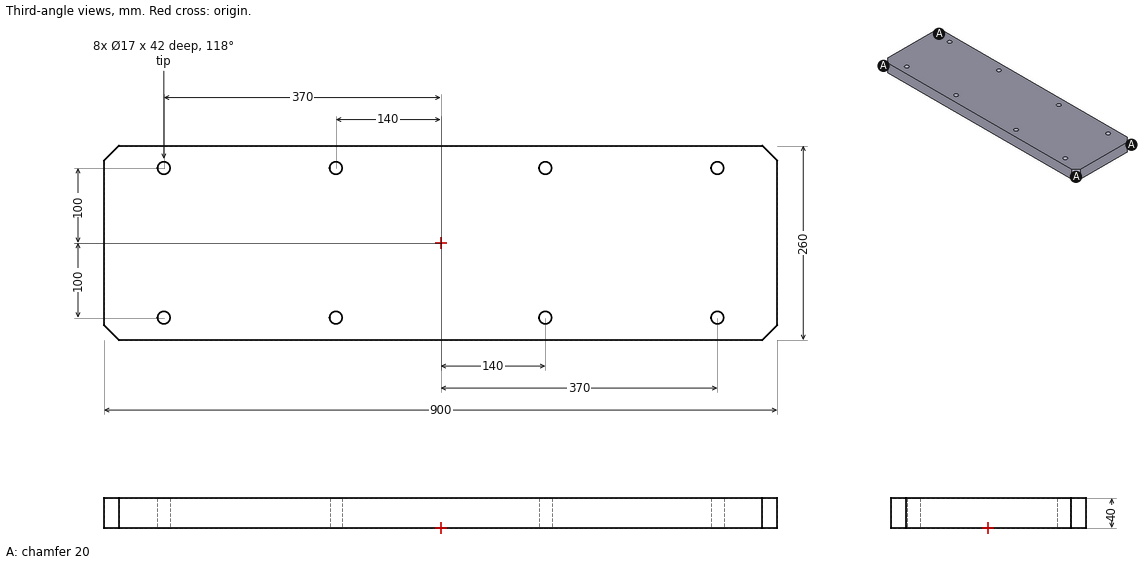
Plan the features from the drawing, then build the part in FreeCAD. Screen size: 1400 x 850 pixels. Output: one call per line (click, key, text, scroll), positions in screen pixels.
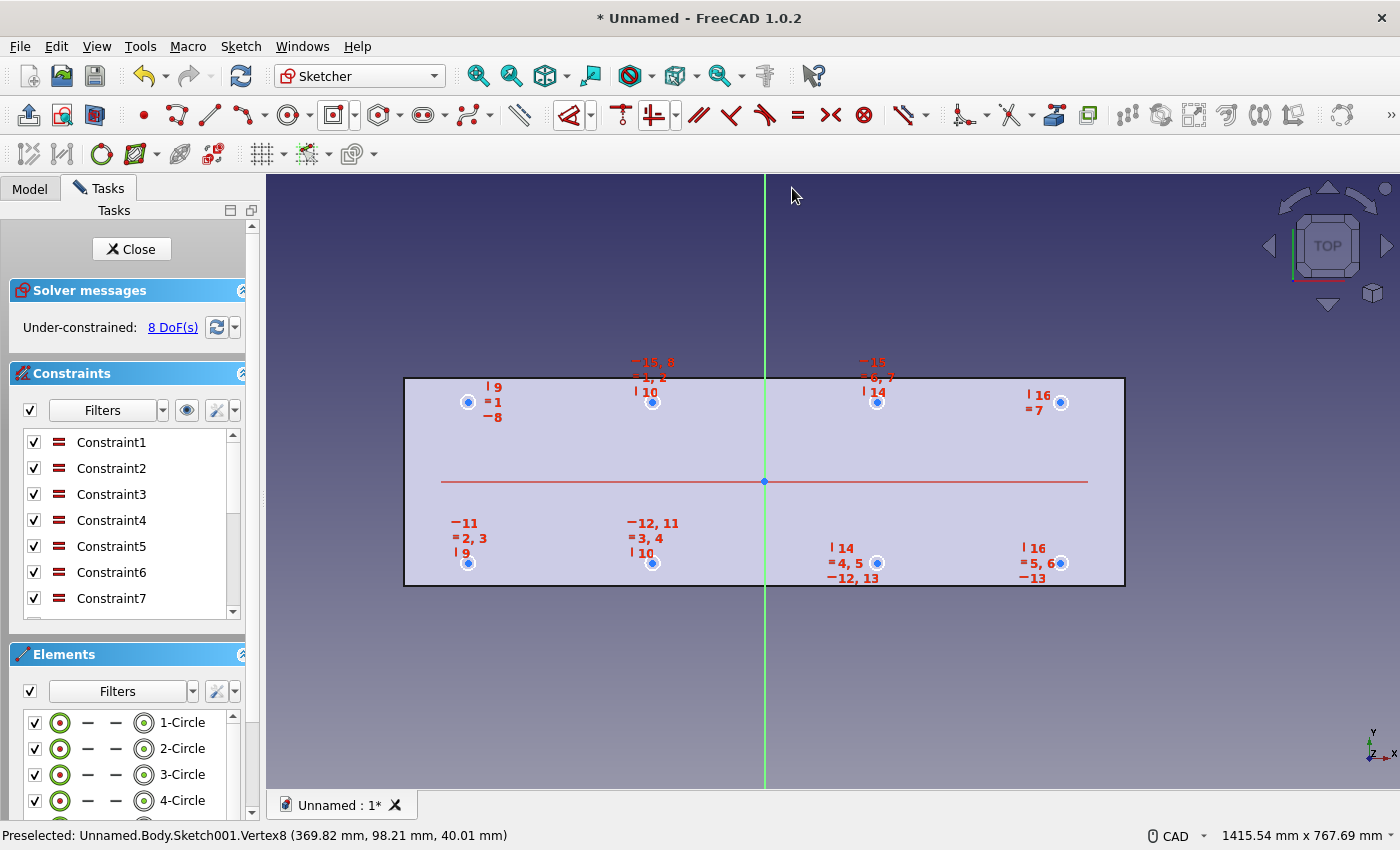
click(877, 402)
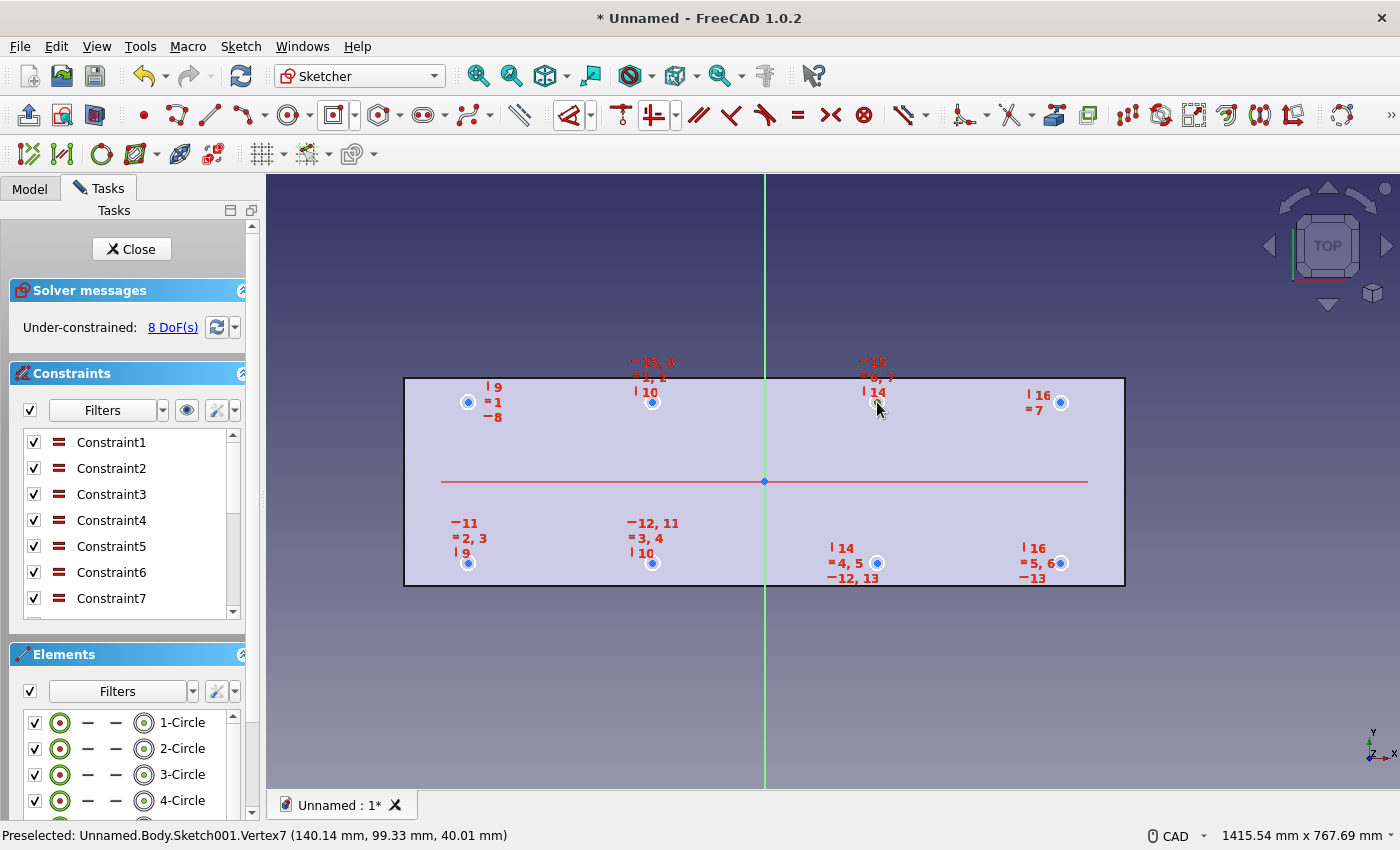
click(1061, 403)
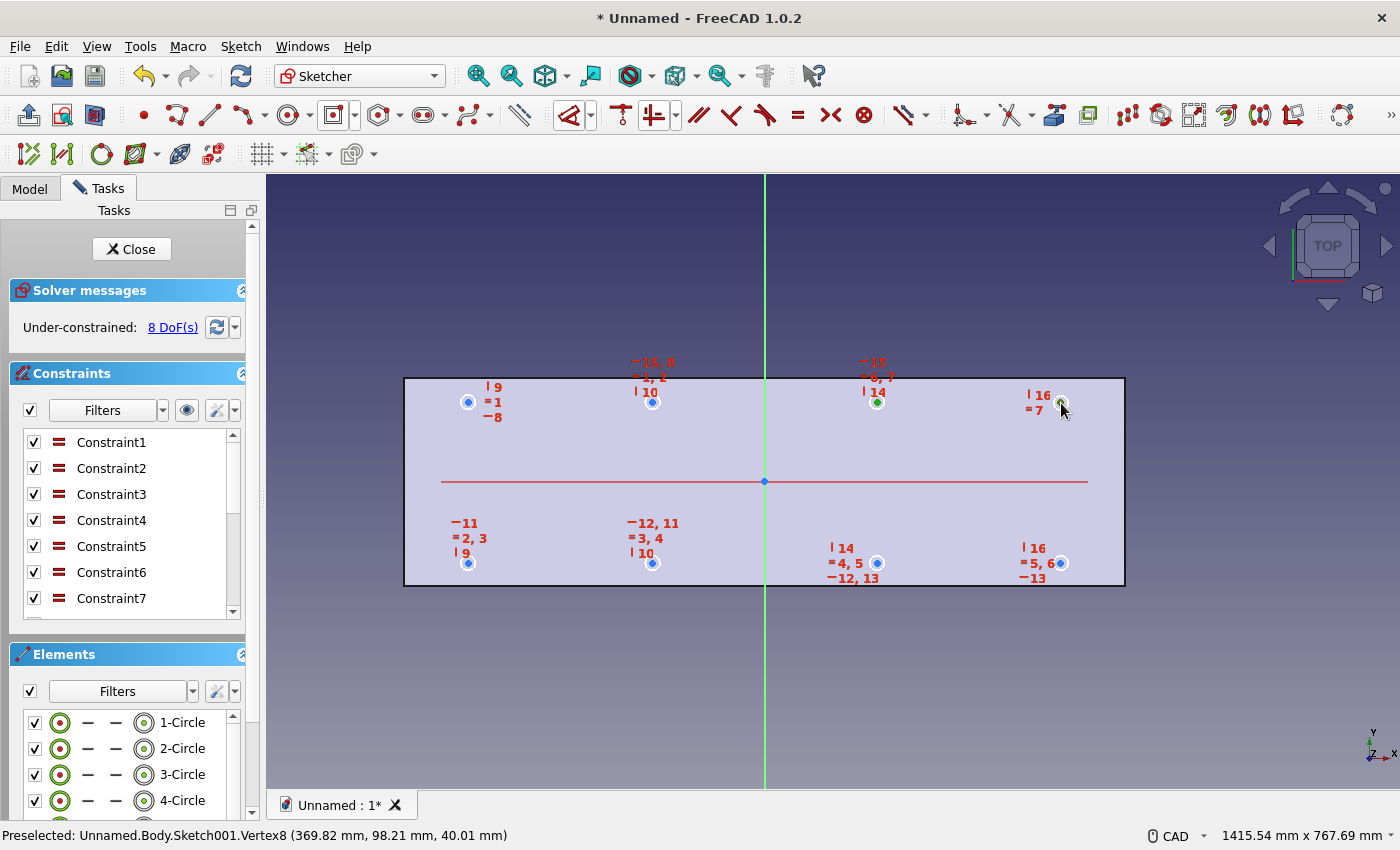
key(h)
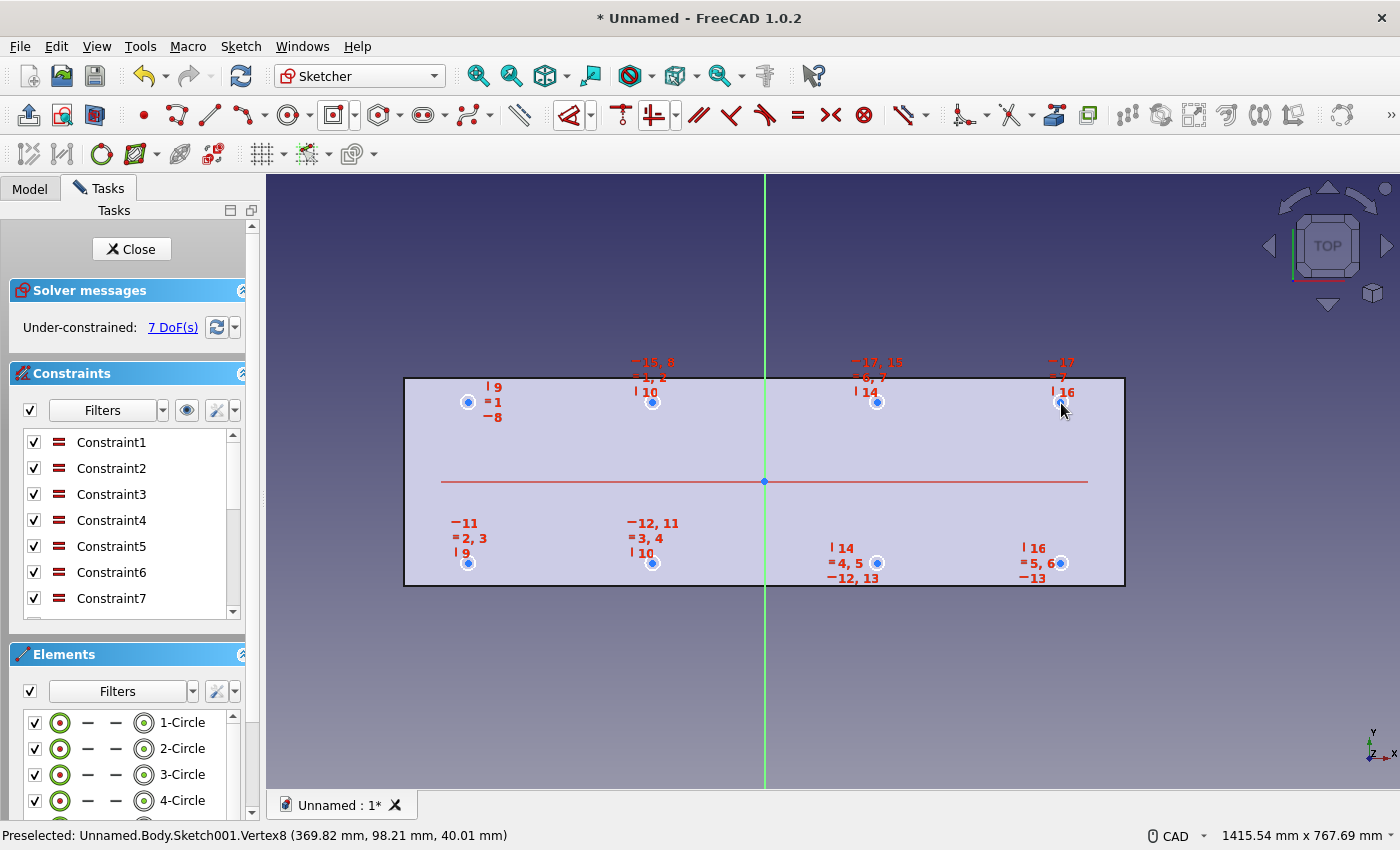
scroll(468, 395, up, 6)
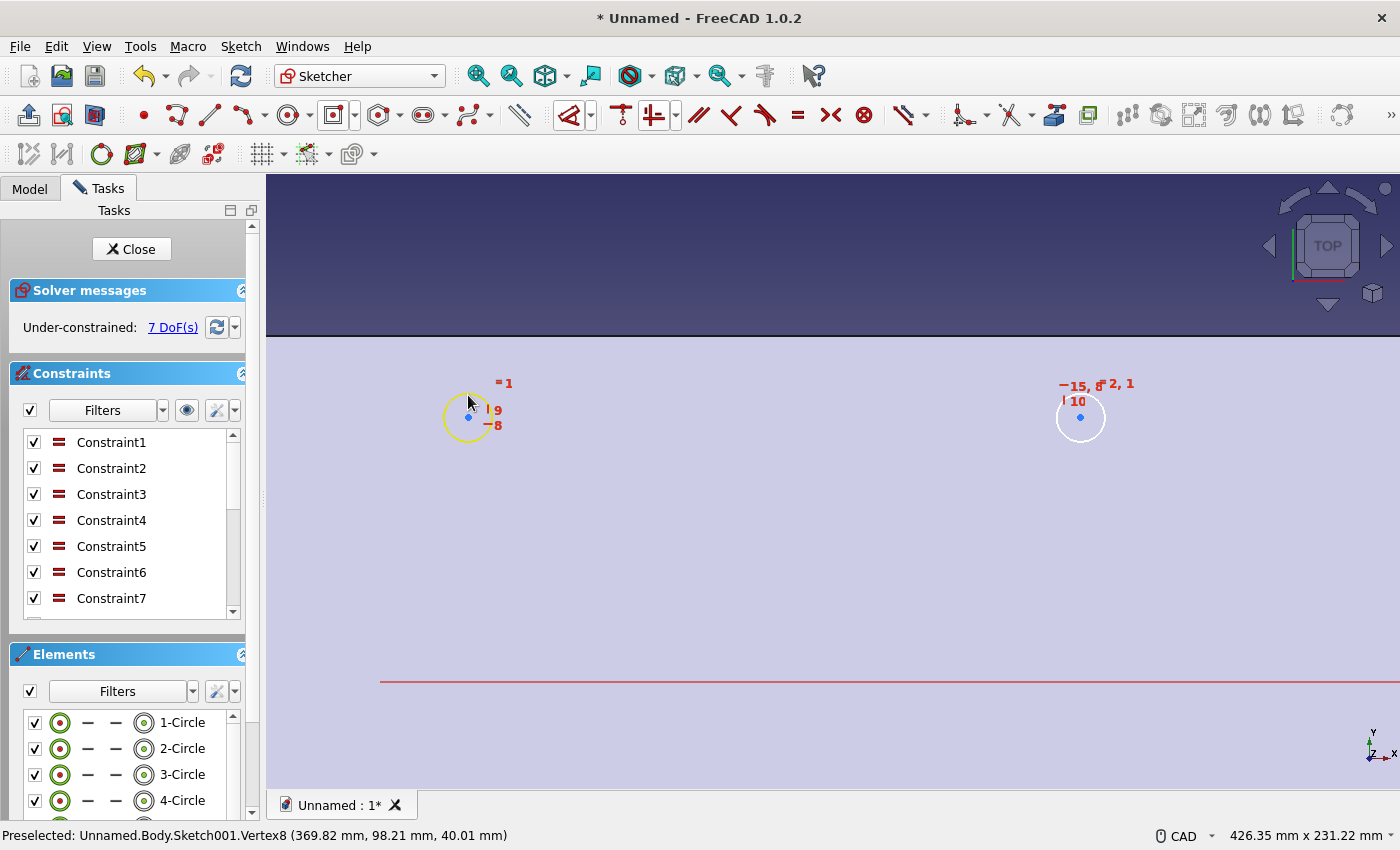
click(469, 394)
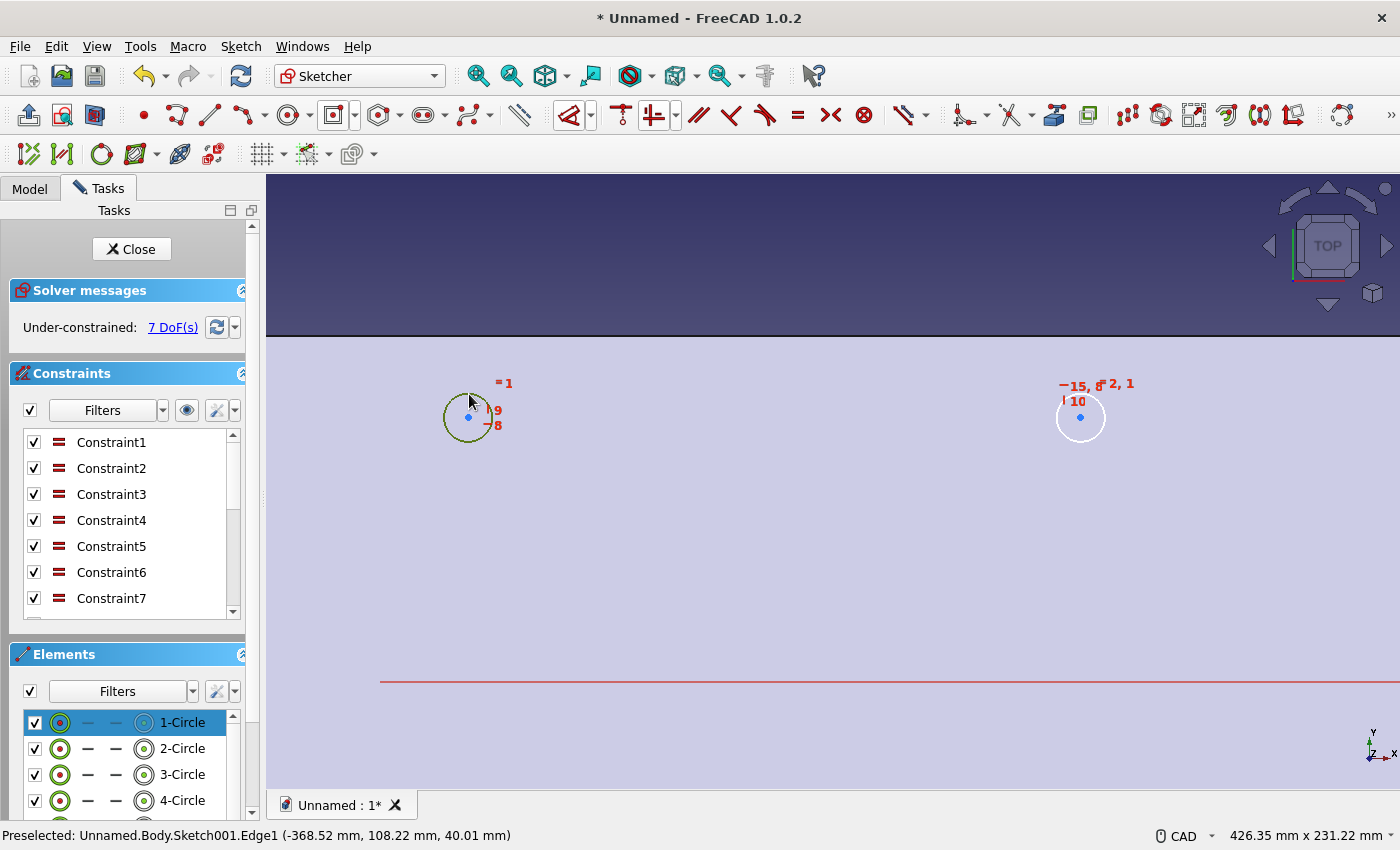
click(590, 116)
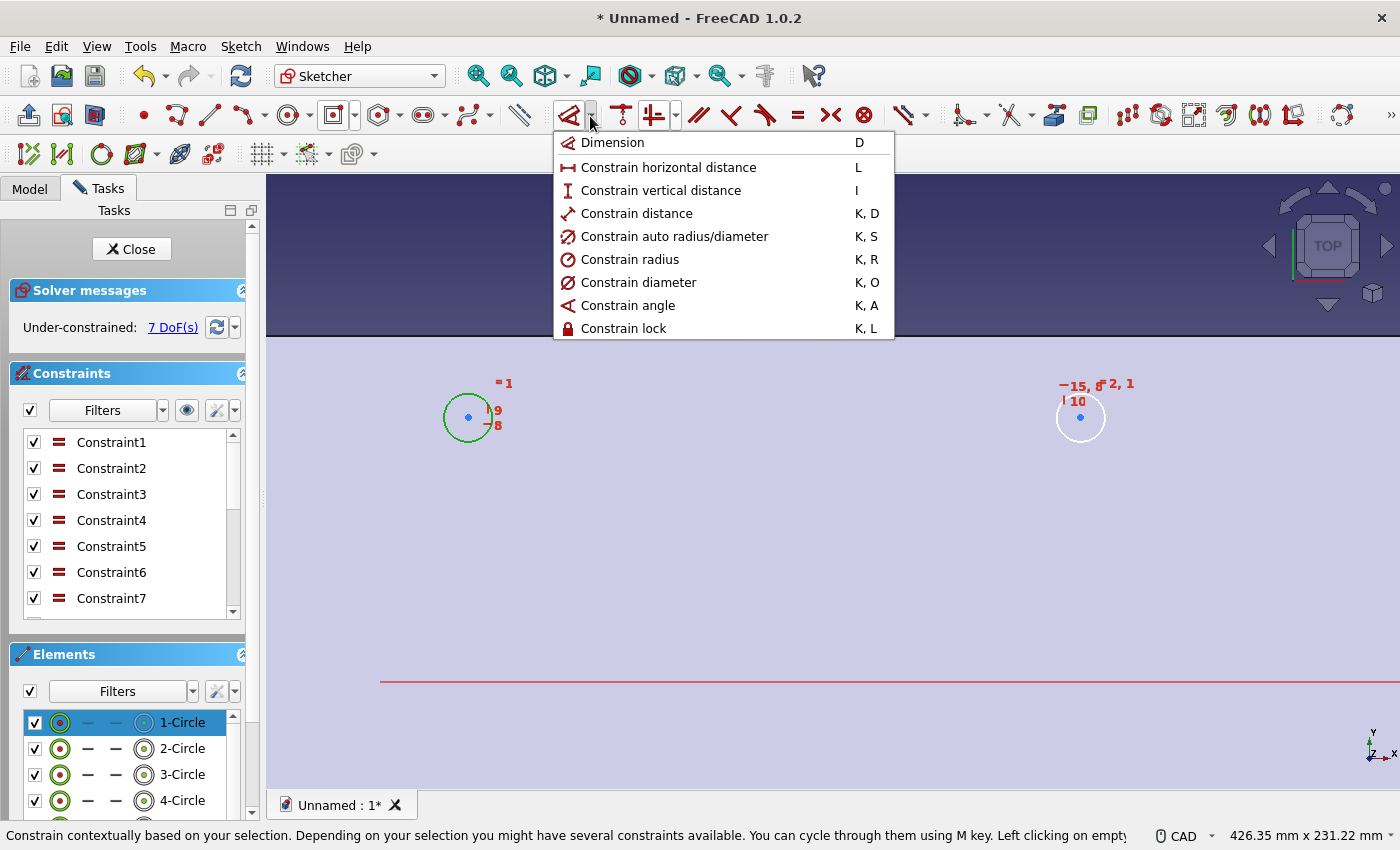
click(724, 282)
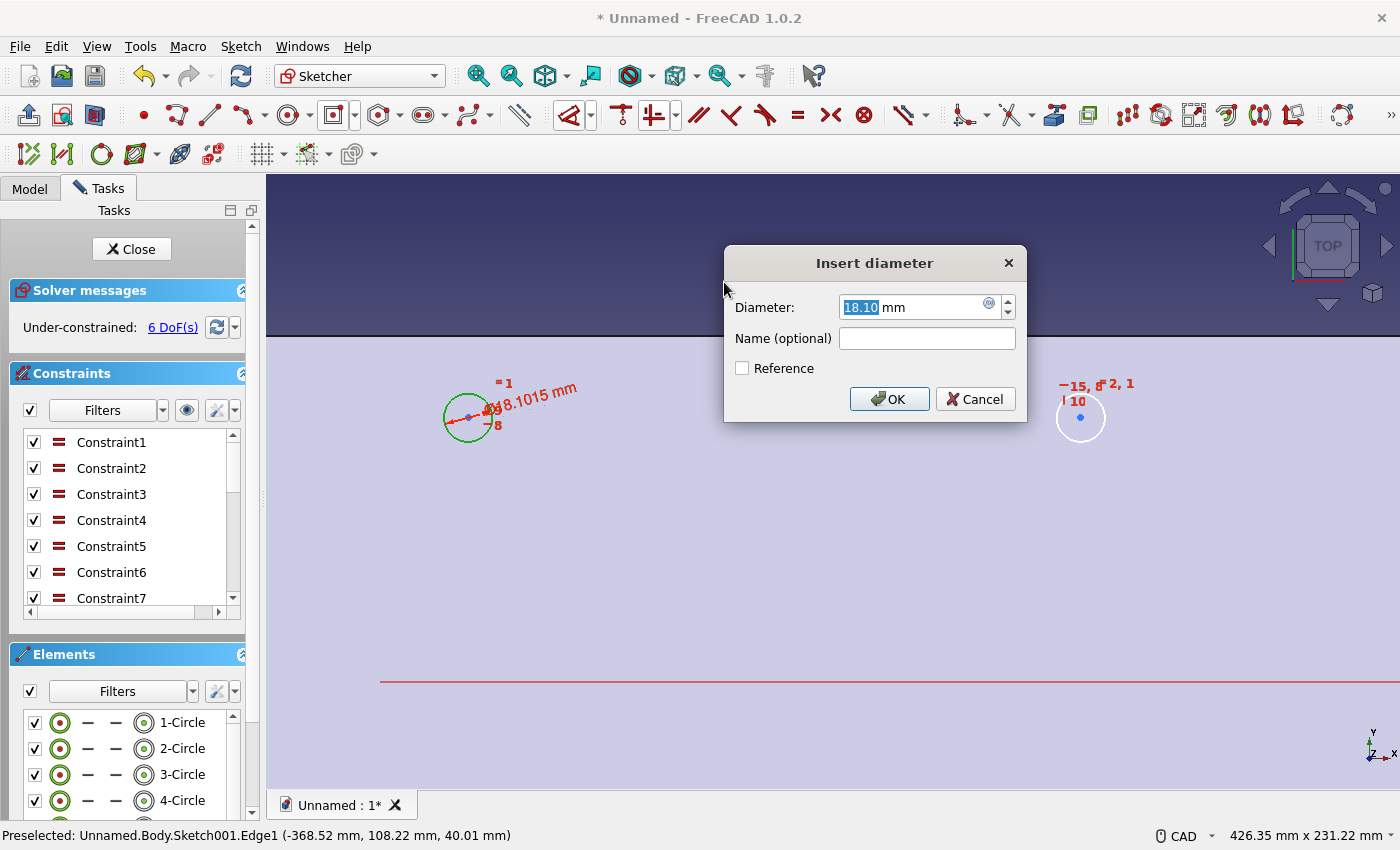
text(17)
key(Return)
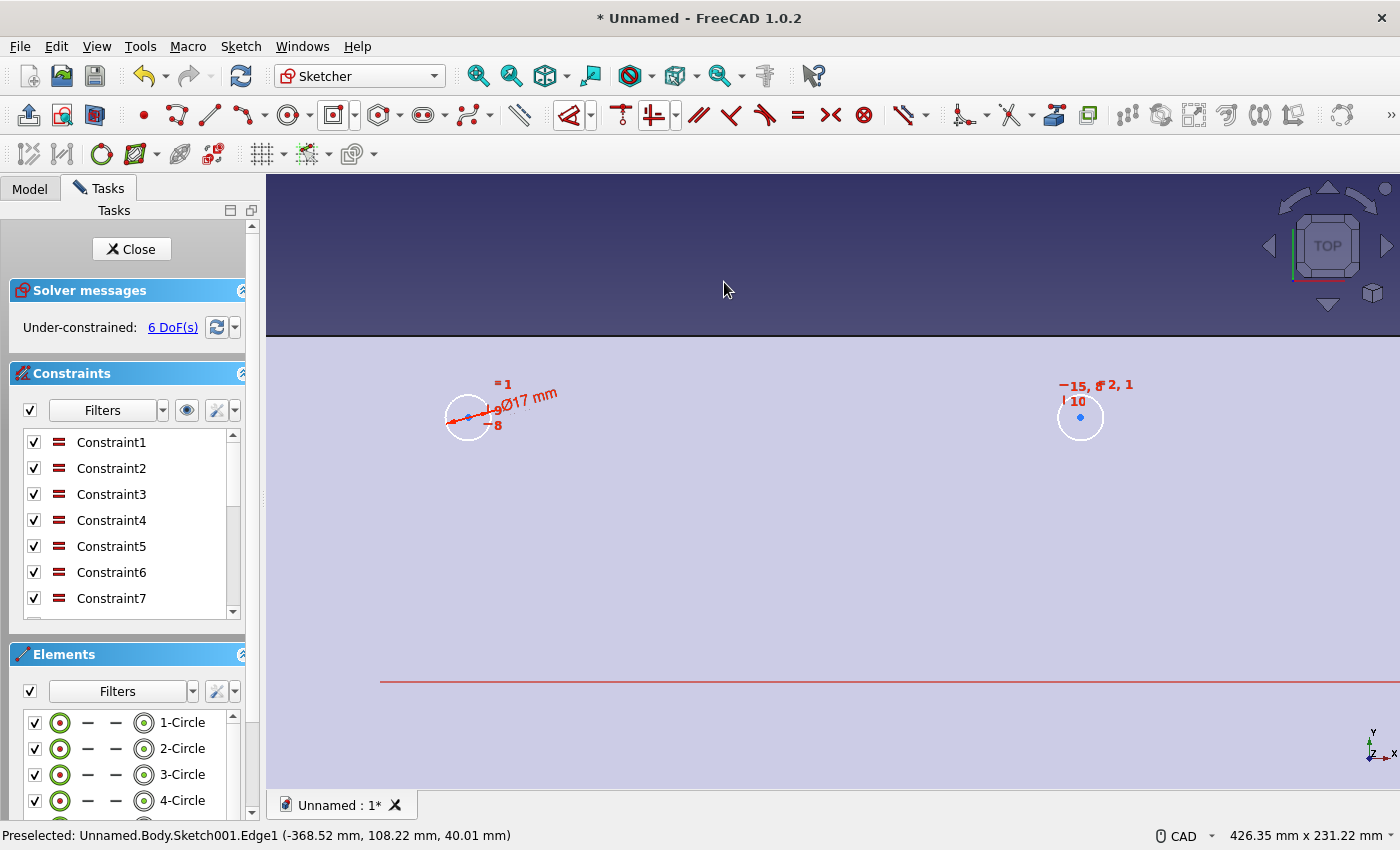
scroll(468, 395, down, 6)